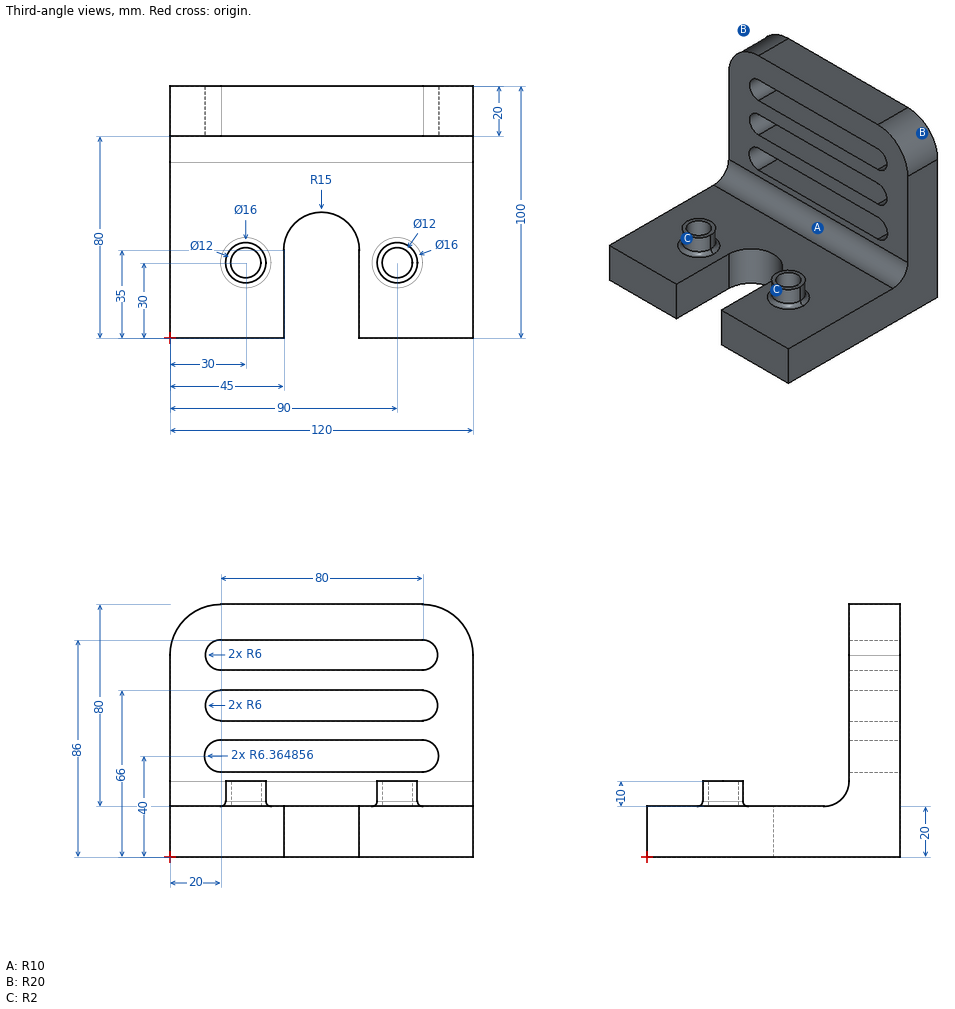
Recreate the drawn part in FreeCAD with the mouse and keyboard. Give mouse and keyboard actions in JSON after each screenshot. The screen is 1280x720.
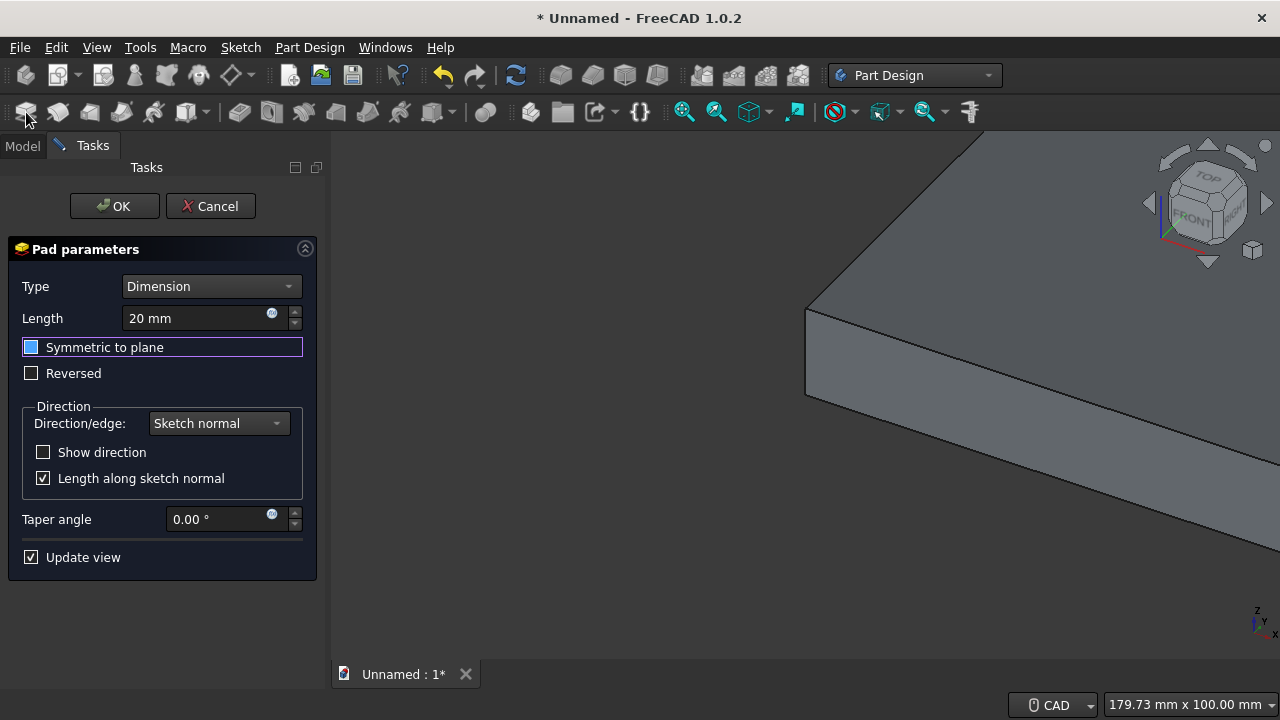
{"action": "left_click", "coordinate": [115, 206]}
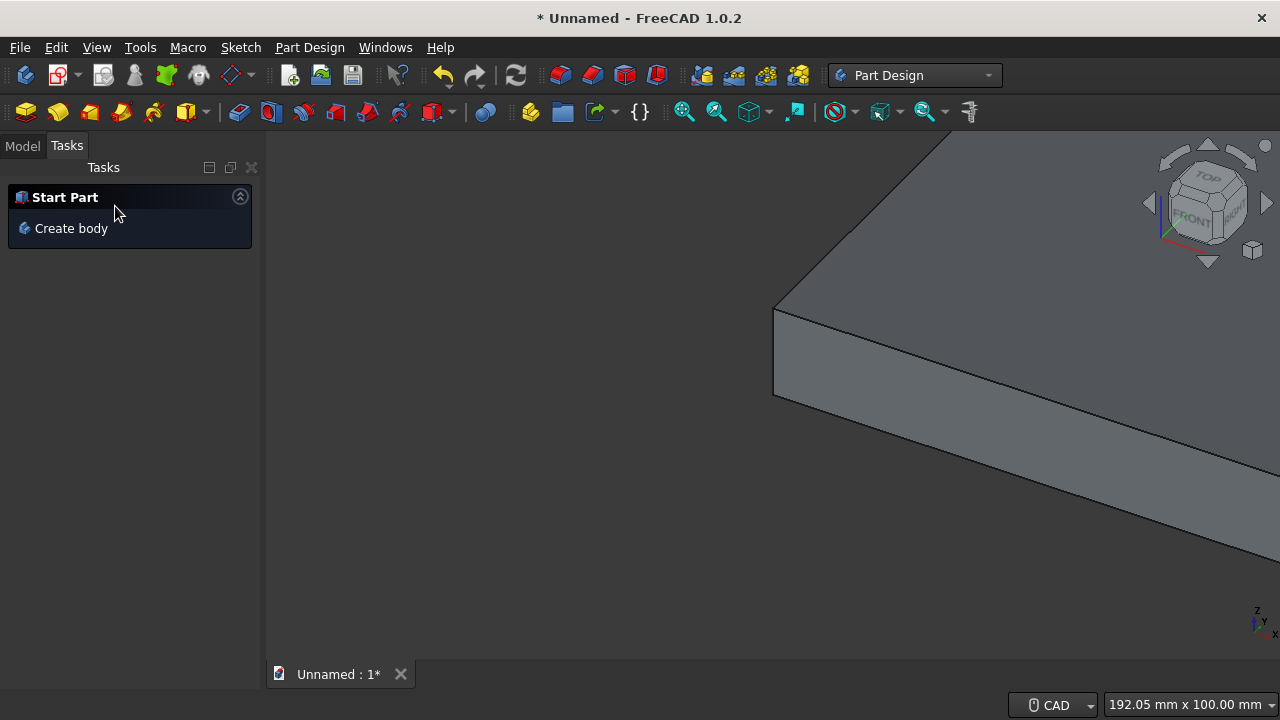
{"action": "left_click", "coordinate": [686, 112]}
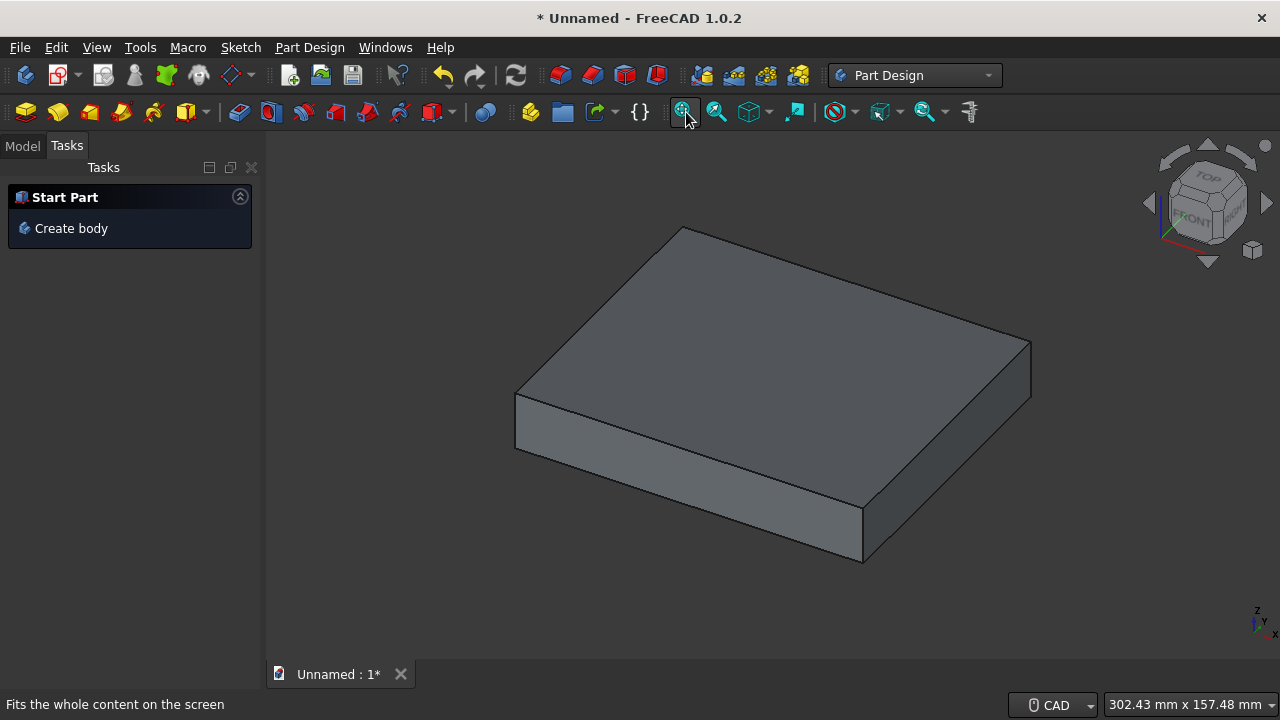
{"action": "left_click", "coordinate": [773, 367]}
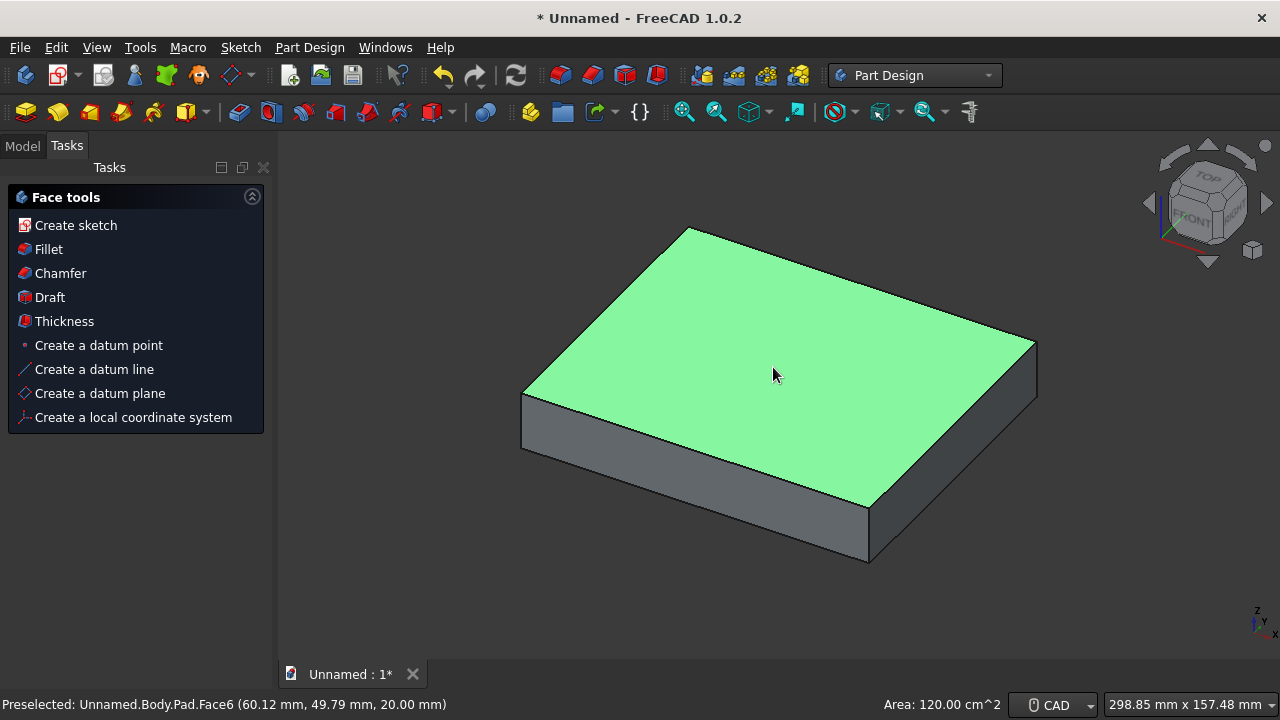
{"action": "left_click", "coordinate": [58, 76]}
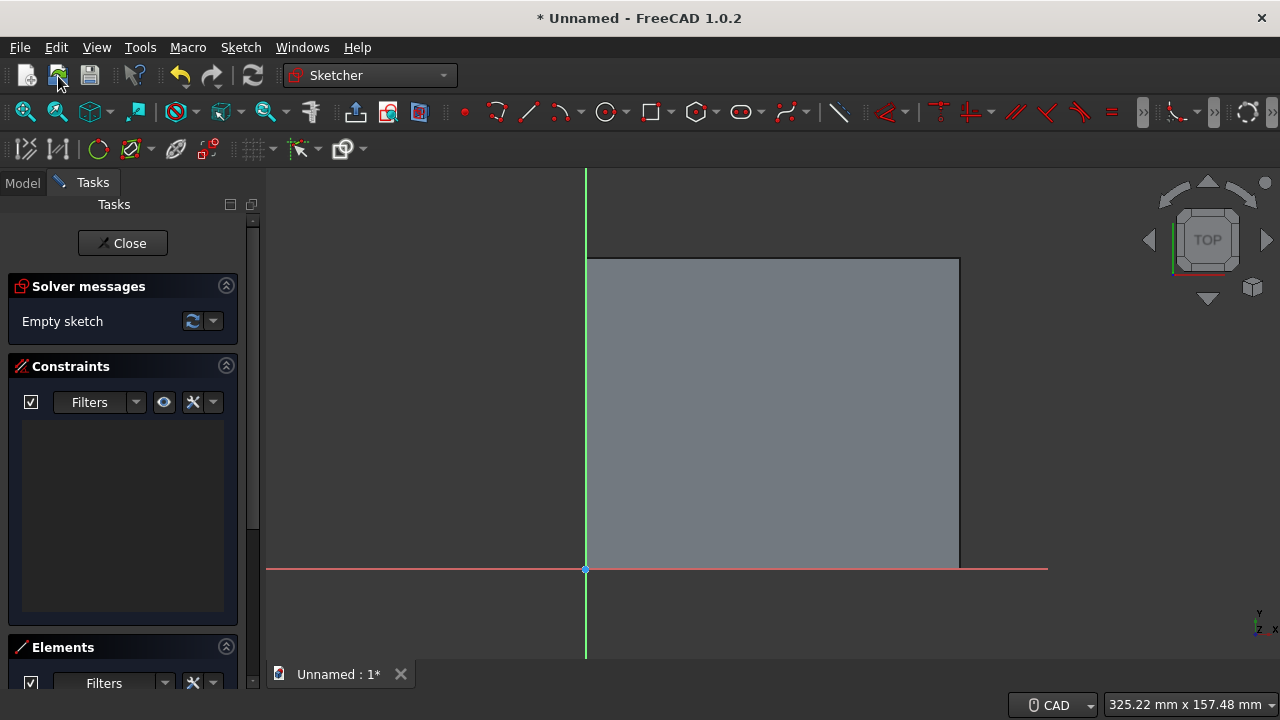
{"action": "left_click", "coordinate": [652, 112]}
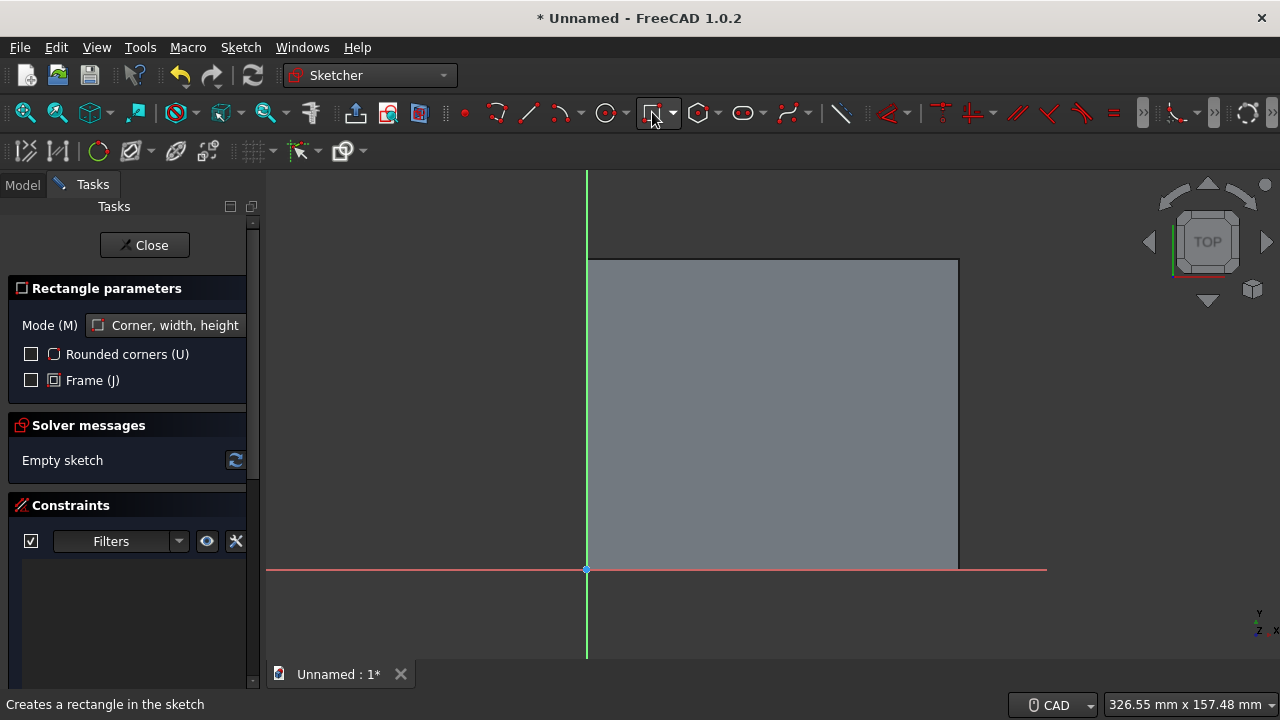
{"action": "left_click", "coordinate": [587, 259]}
{"action": "mouse_move", "coordinate": [959, 321]}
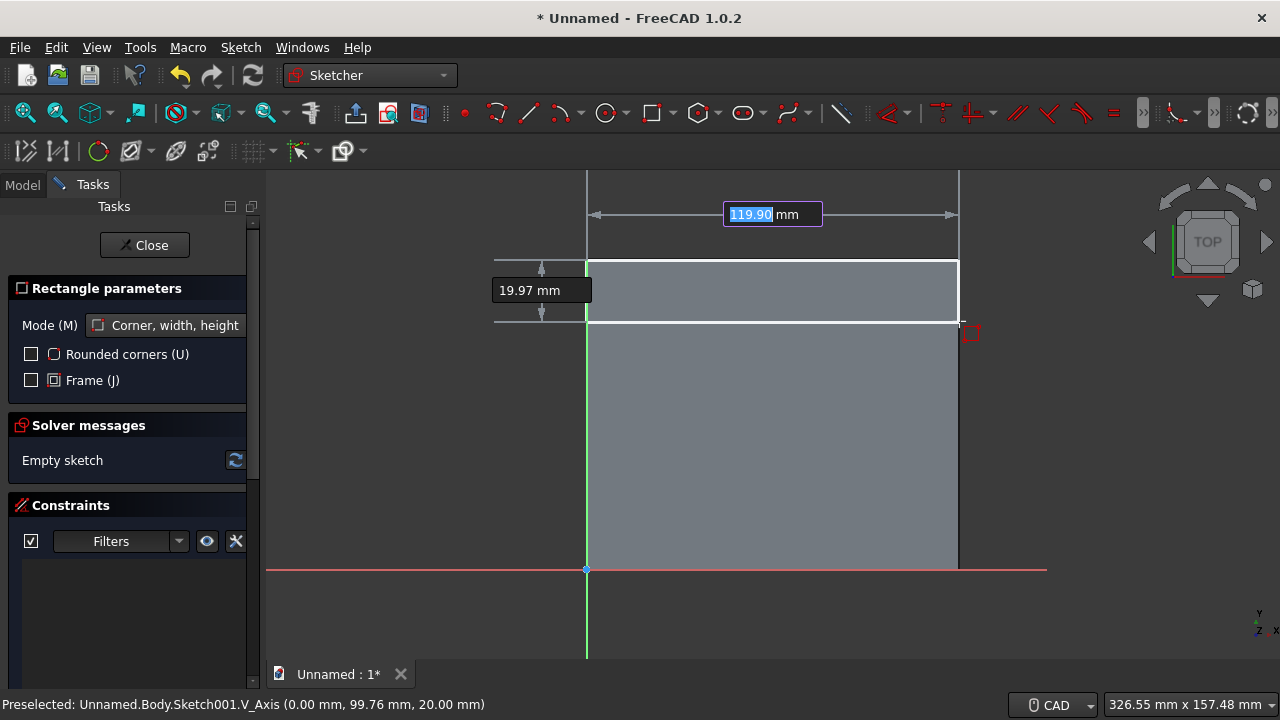
{"action": "type", "text": "120"}
{"action": "key", "text": "Tab"}
{"action": "type", "text": "20"}
{"action": "key", "text": "Return"}
{"action": "key", "text": "Escape"}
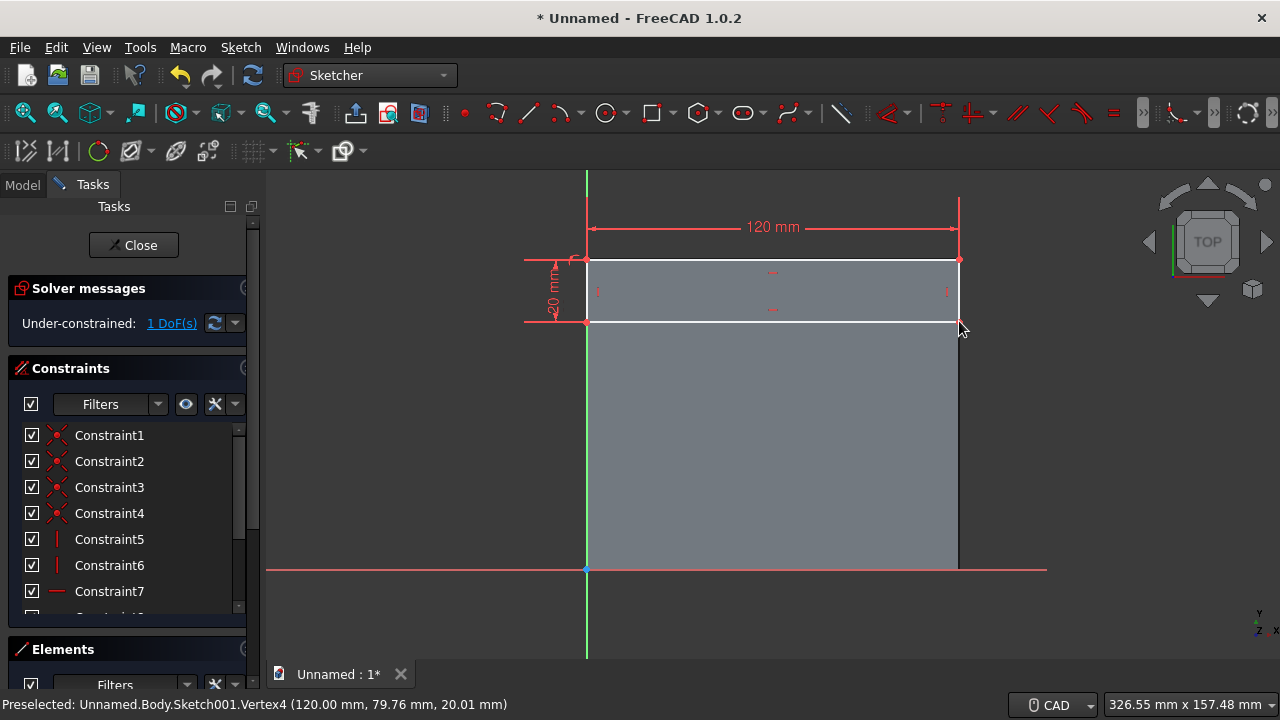
{"action": "left_click", "coordinate": [888, 114]}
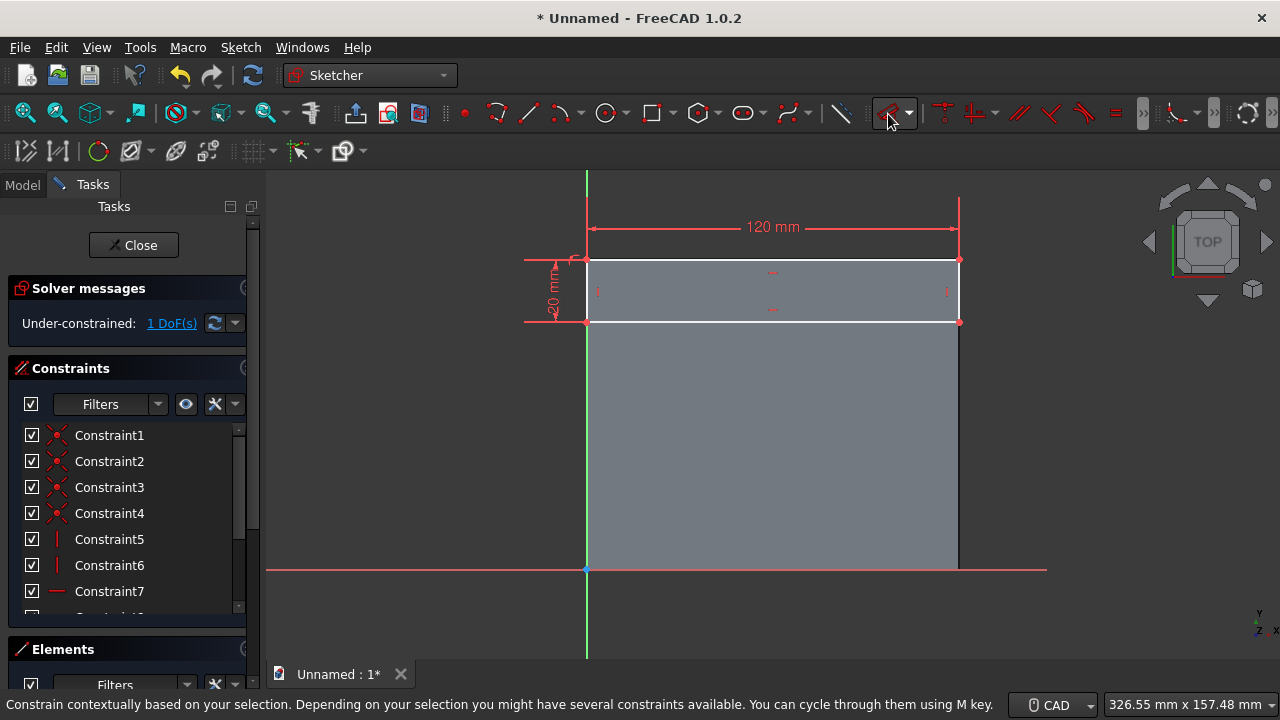
{"action": "left_click", "coordinate": [587, 322]}
{"action": "left_click", "coordinate": [553, 446]}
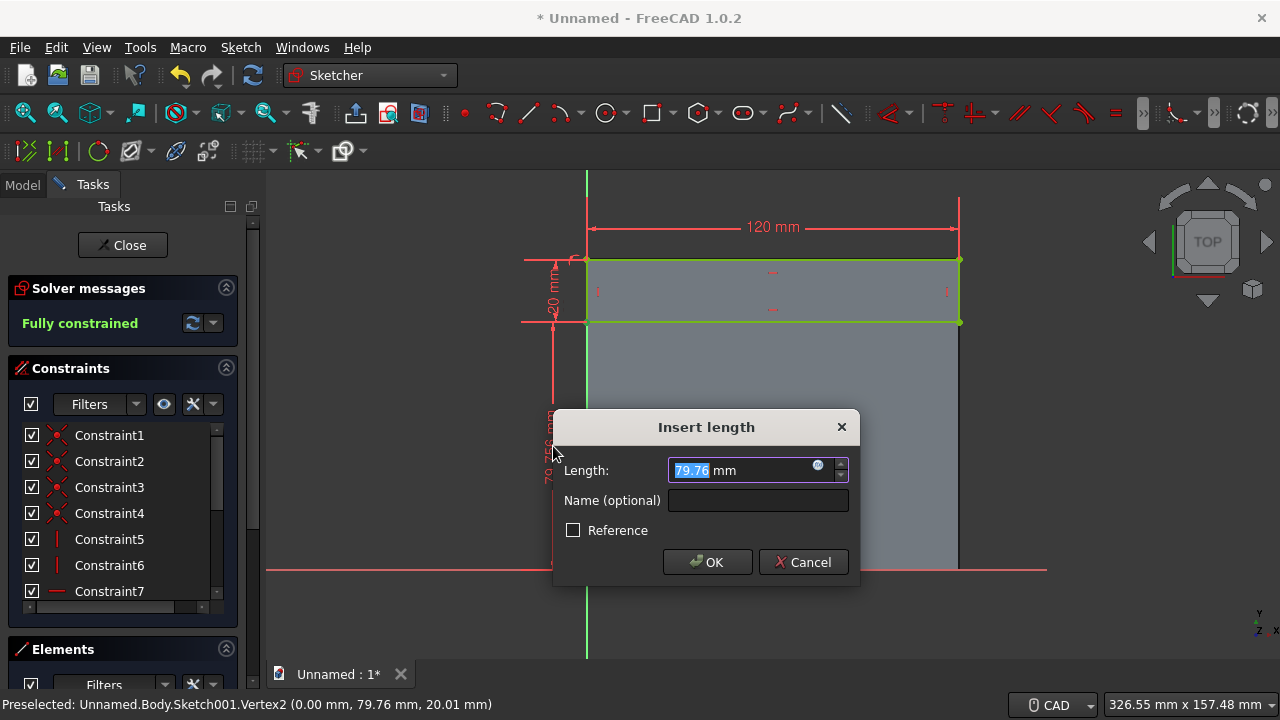
{"action": "type", "text": "80"}
{"action": "key", "text": "Return"}
{"action": "key", "text": "Escape"}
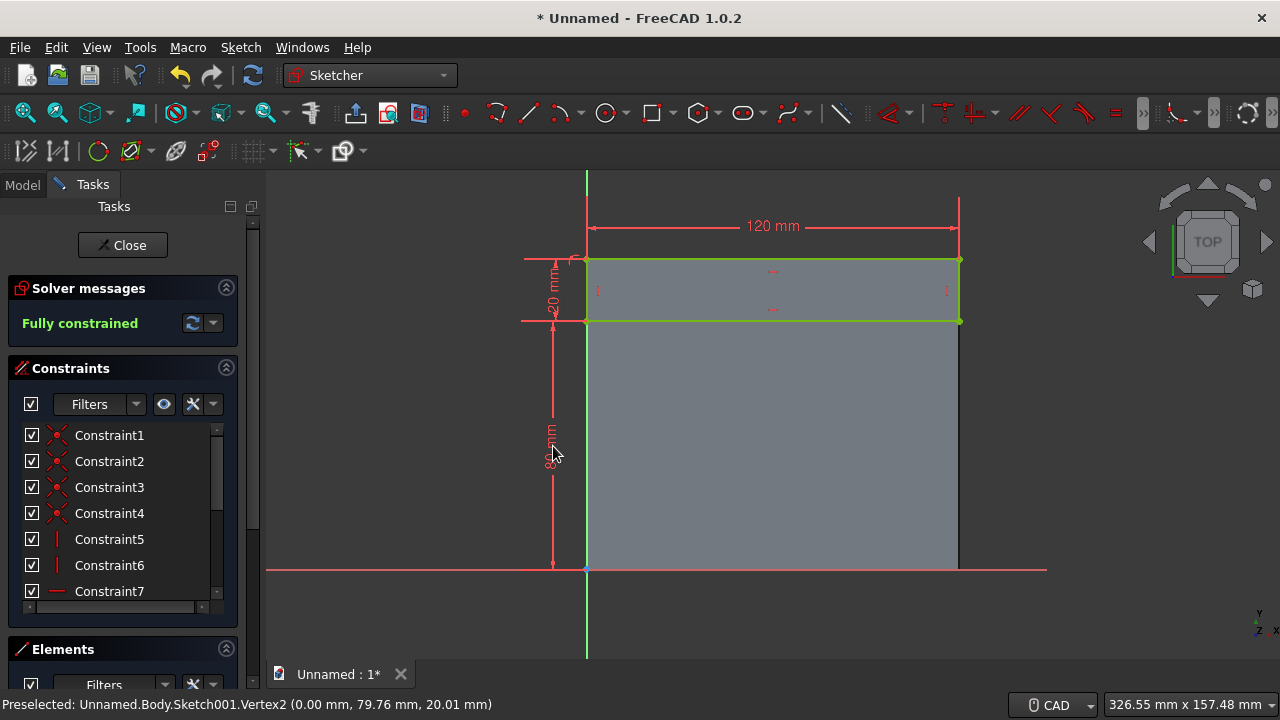
{"action": "left_click", "coordinate": [123, 245]}